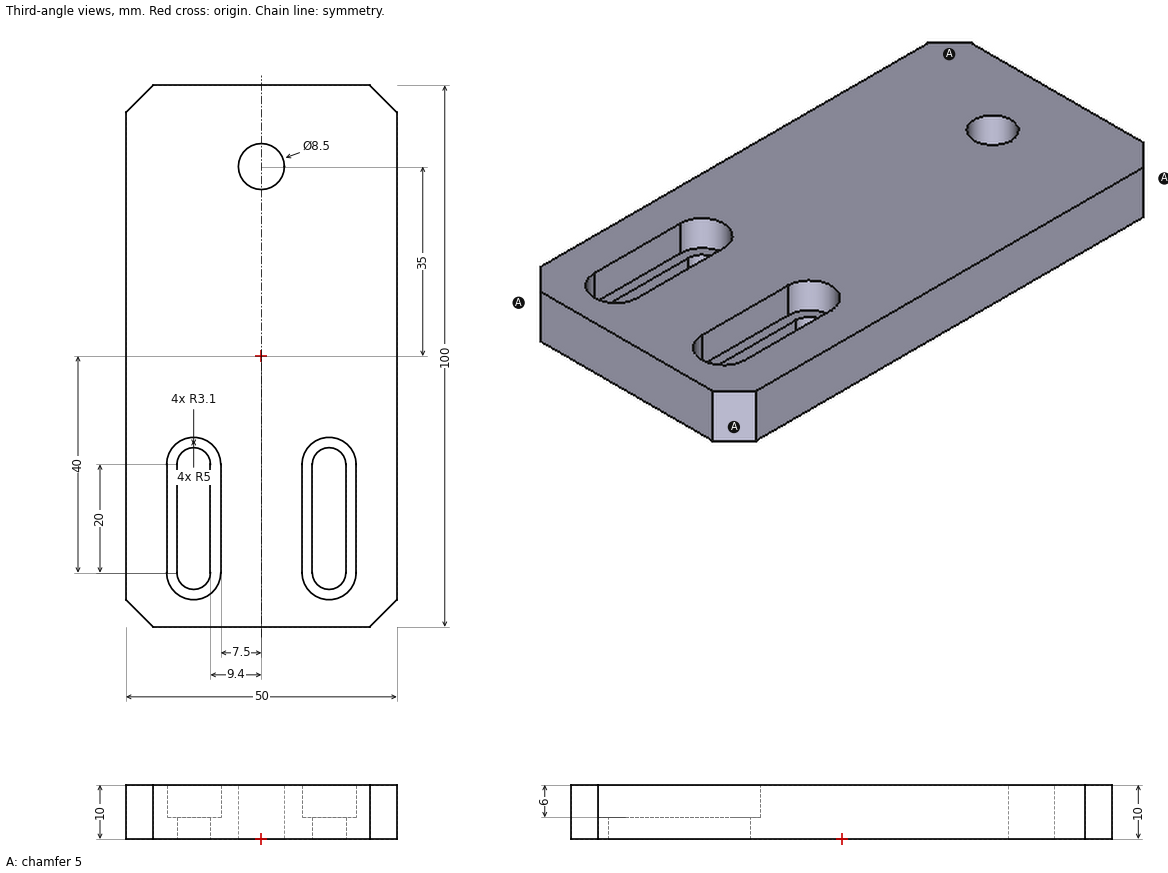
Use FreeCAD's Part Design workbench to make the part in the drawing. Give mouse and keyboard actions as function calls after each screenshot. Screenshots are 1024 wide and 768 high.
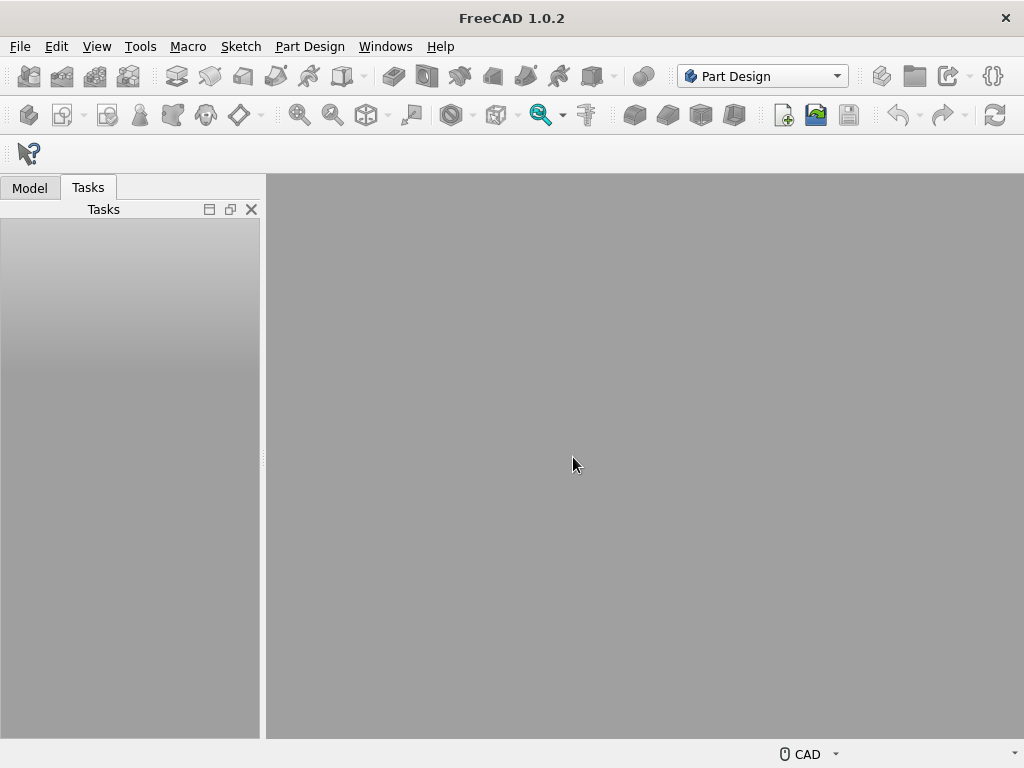
click(783, 116)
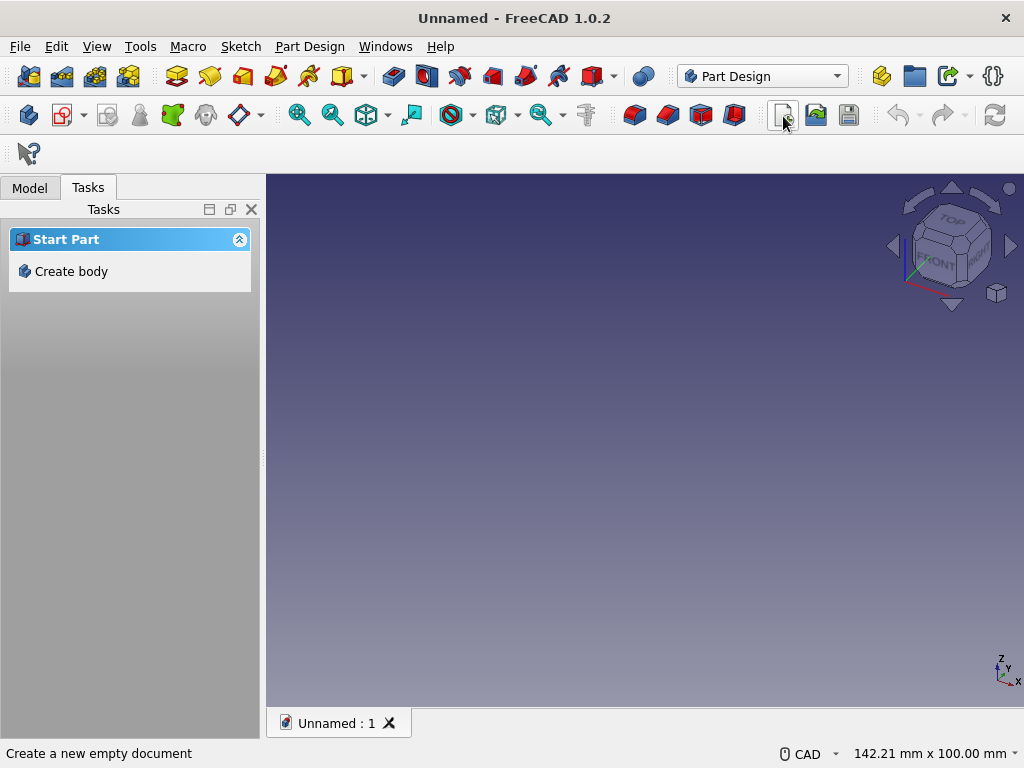
click(62, 116)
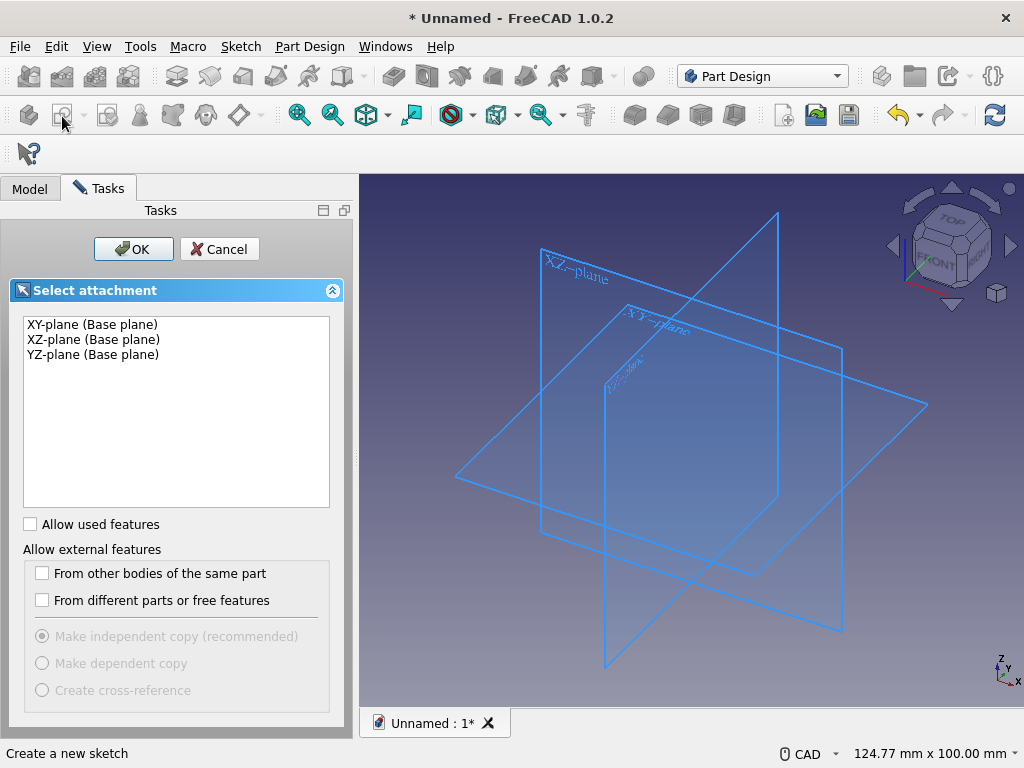
click(84, 324)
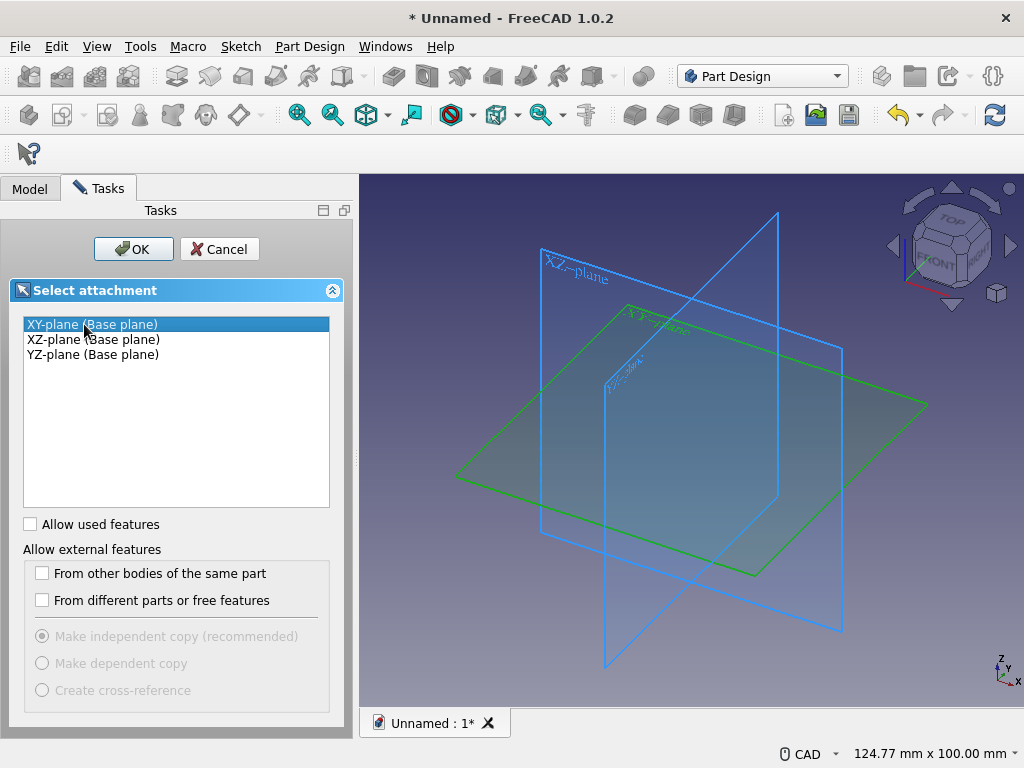
click(134, 249)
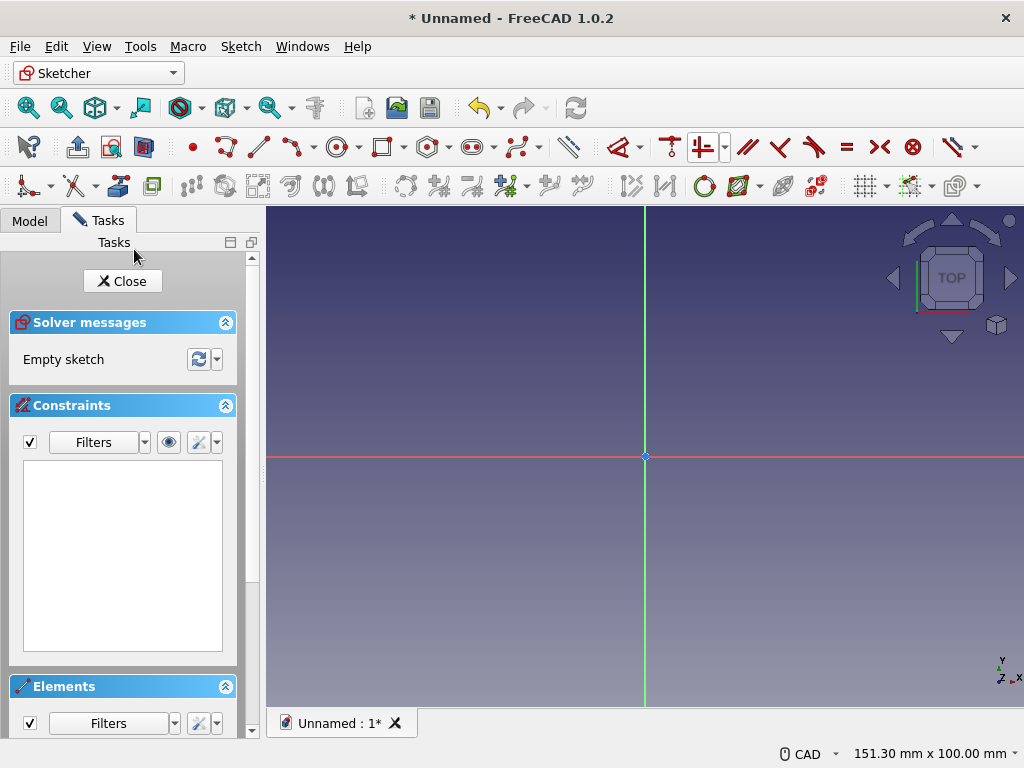
scroll(437, 457, down, 2)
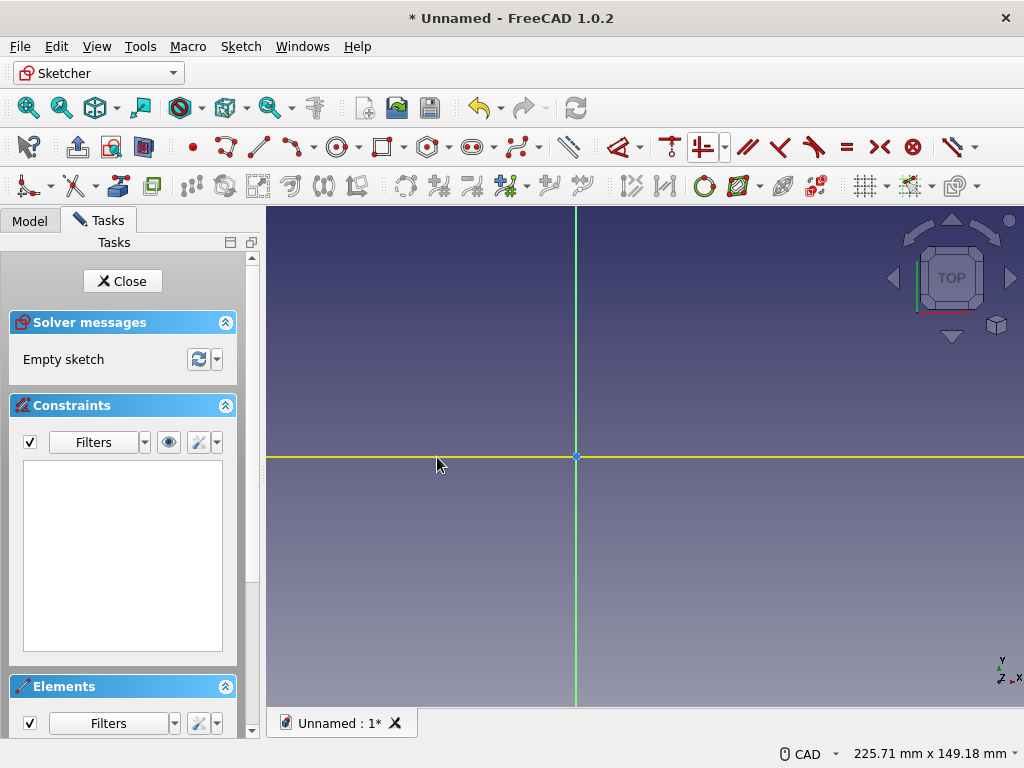
click(404, 148)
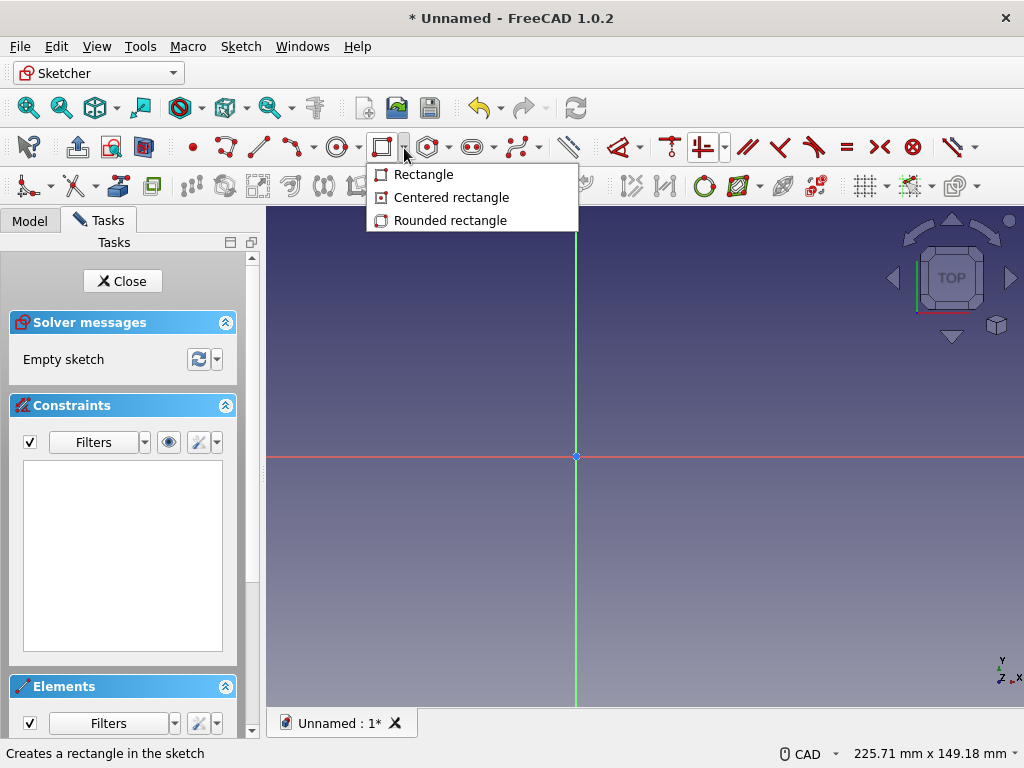
click(472, 198)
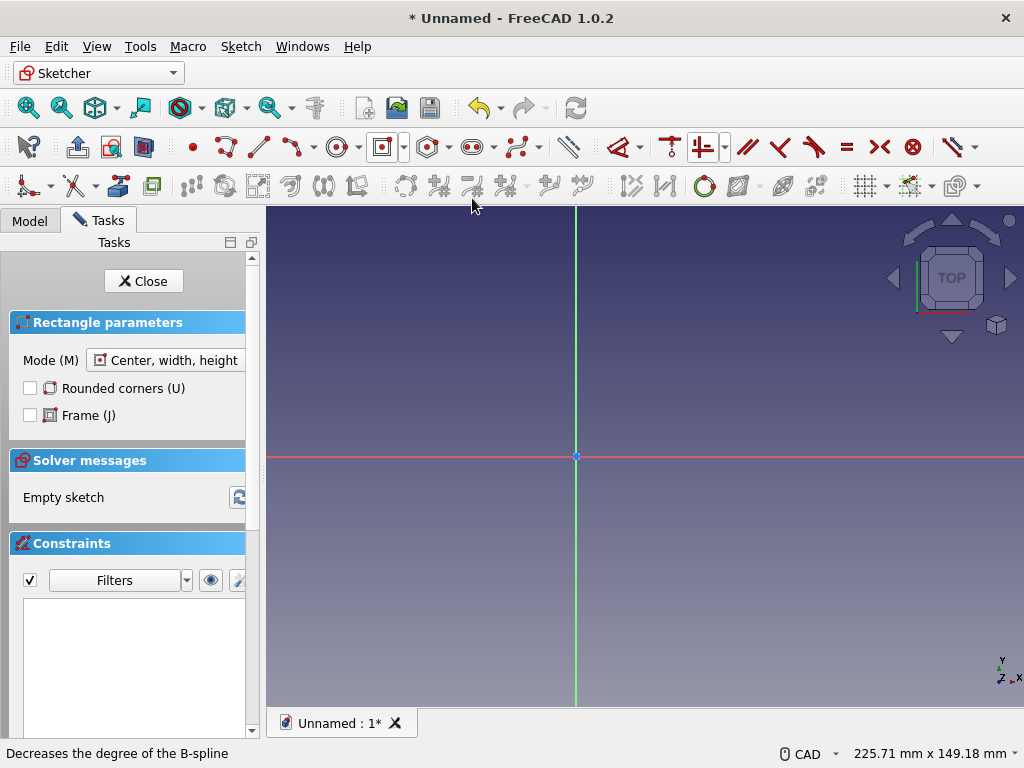
click(577, 457)
click(660, 289)
key(Escape)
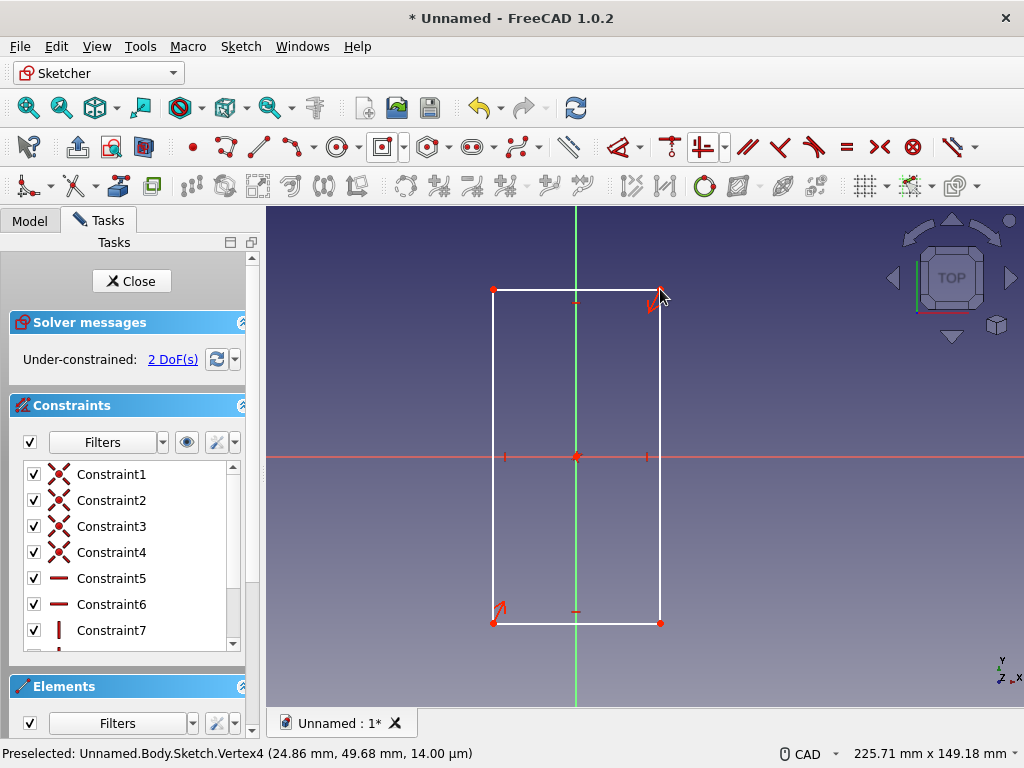
click(543, 624)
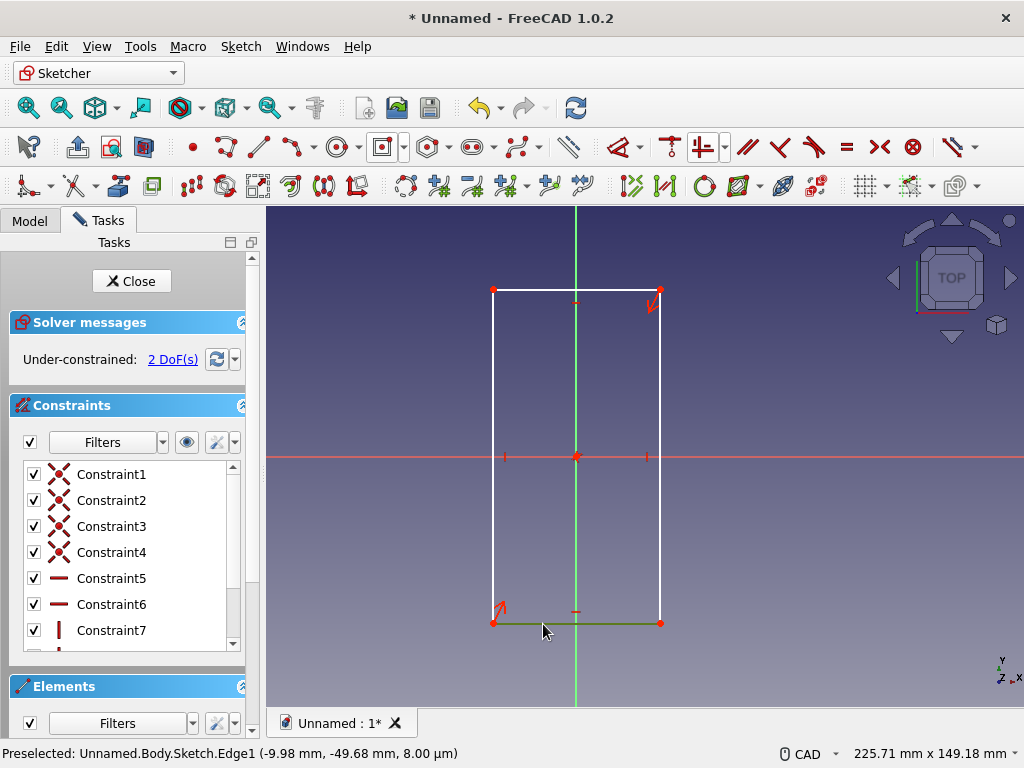
click(640, 148)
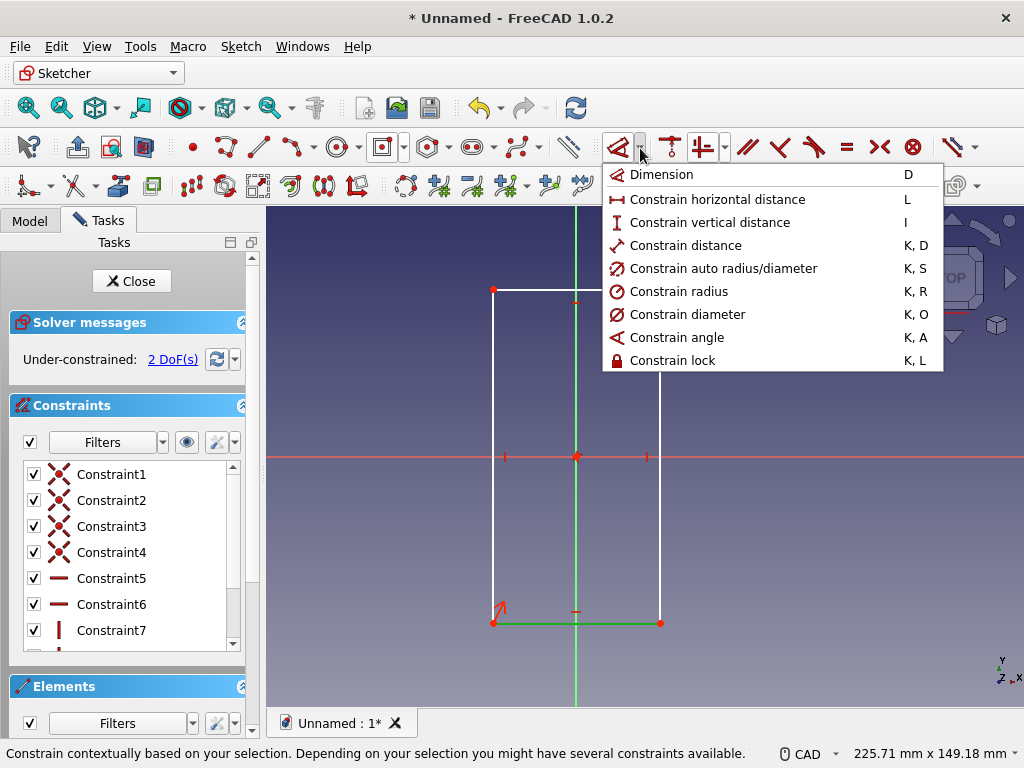
click(773, 200)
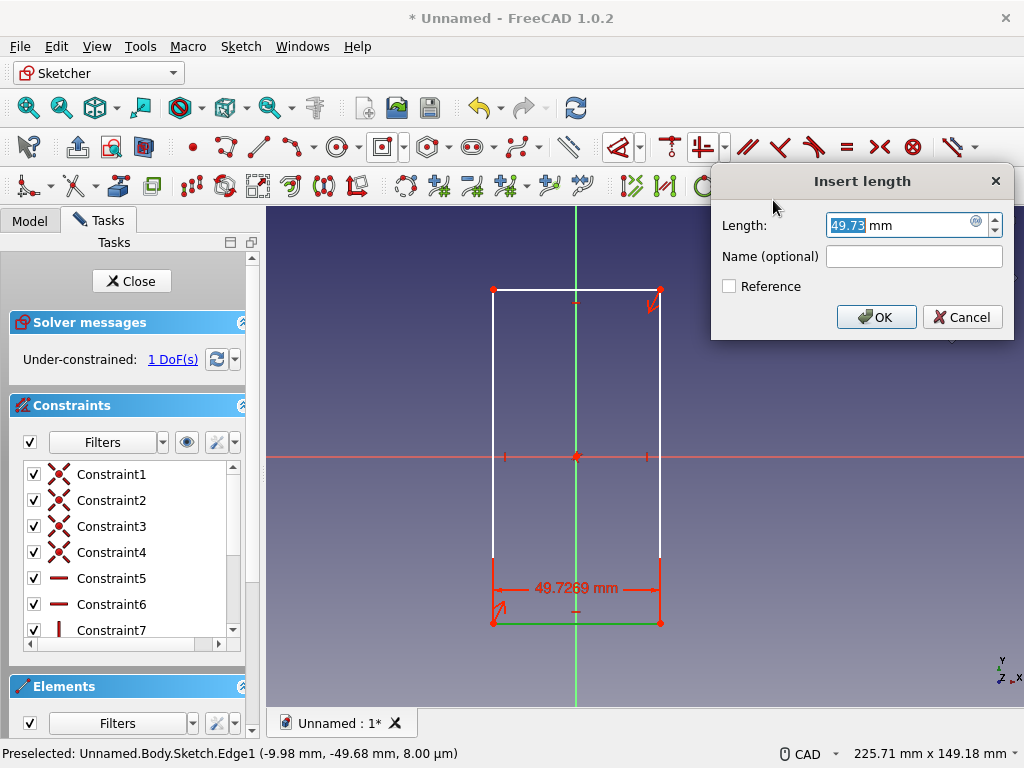
text(50)
key(Return)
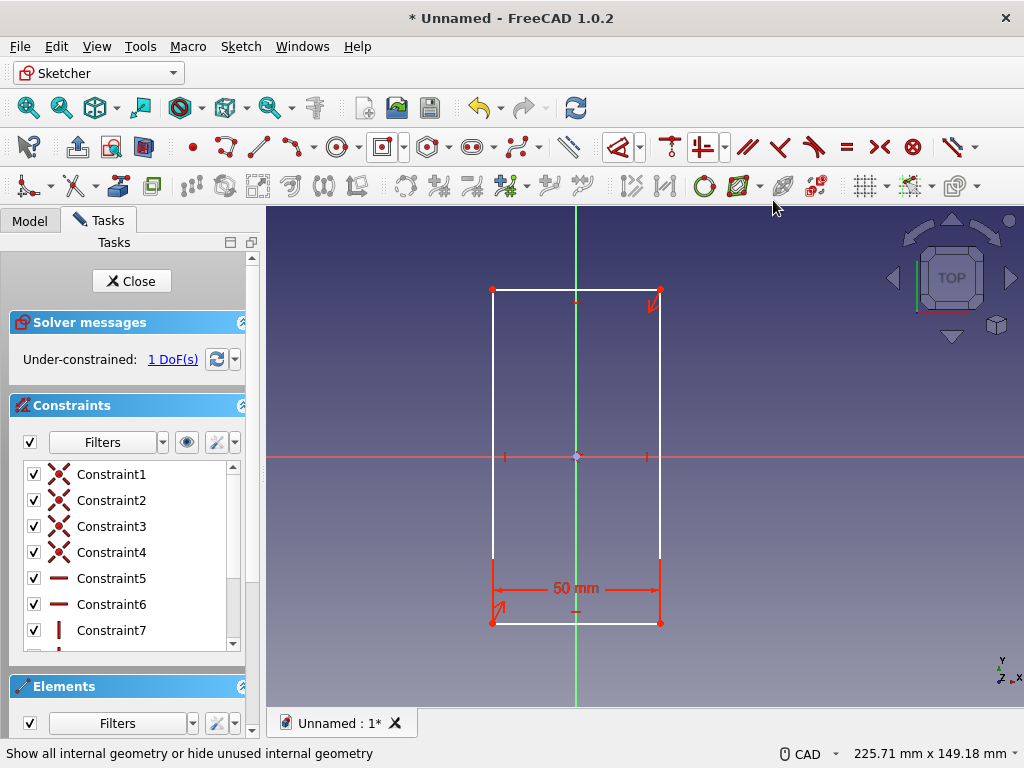
click(660, 524)